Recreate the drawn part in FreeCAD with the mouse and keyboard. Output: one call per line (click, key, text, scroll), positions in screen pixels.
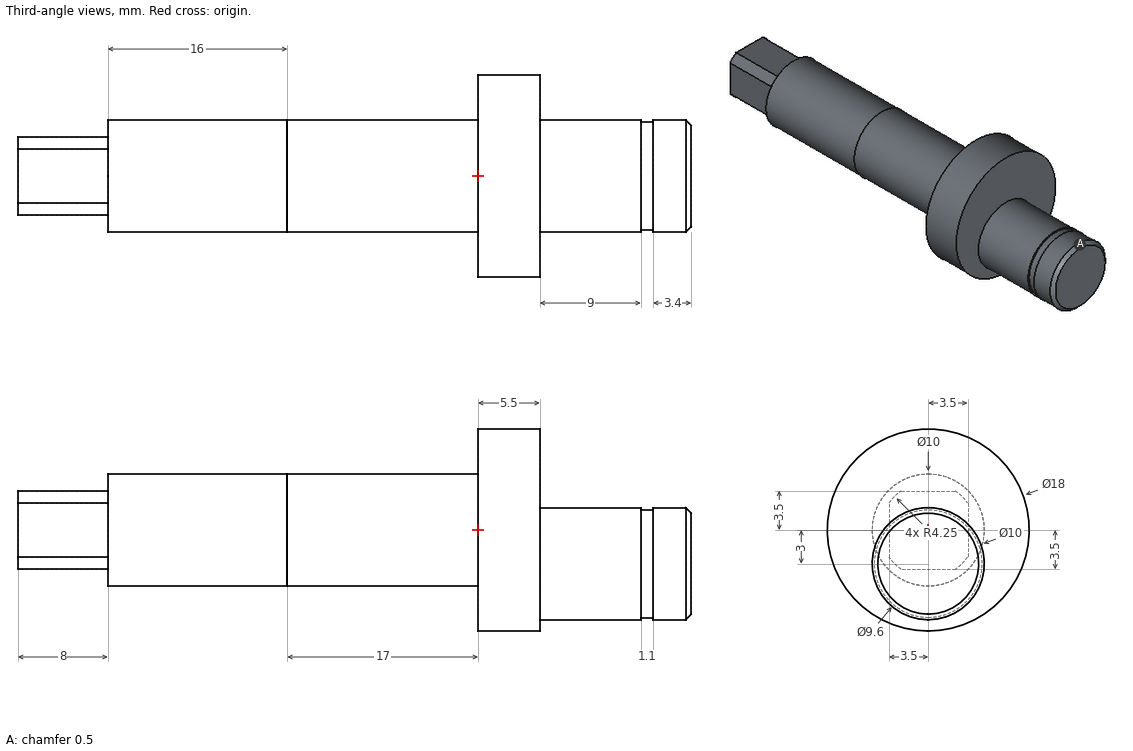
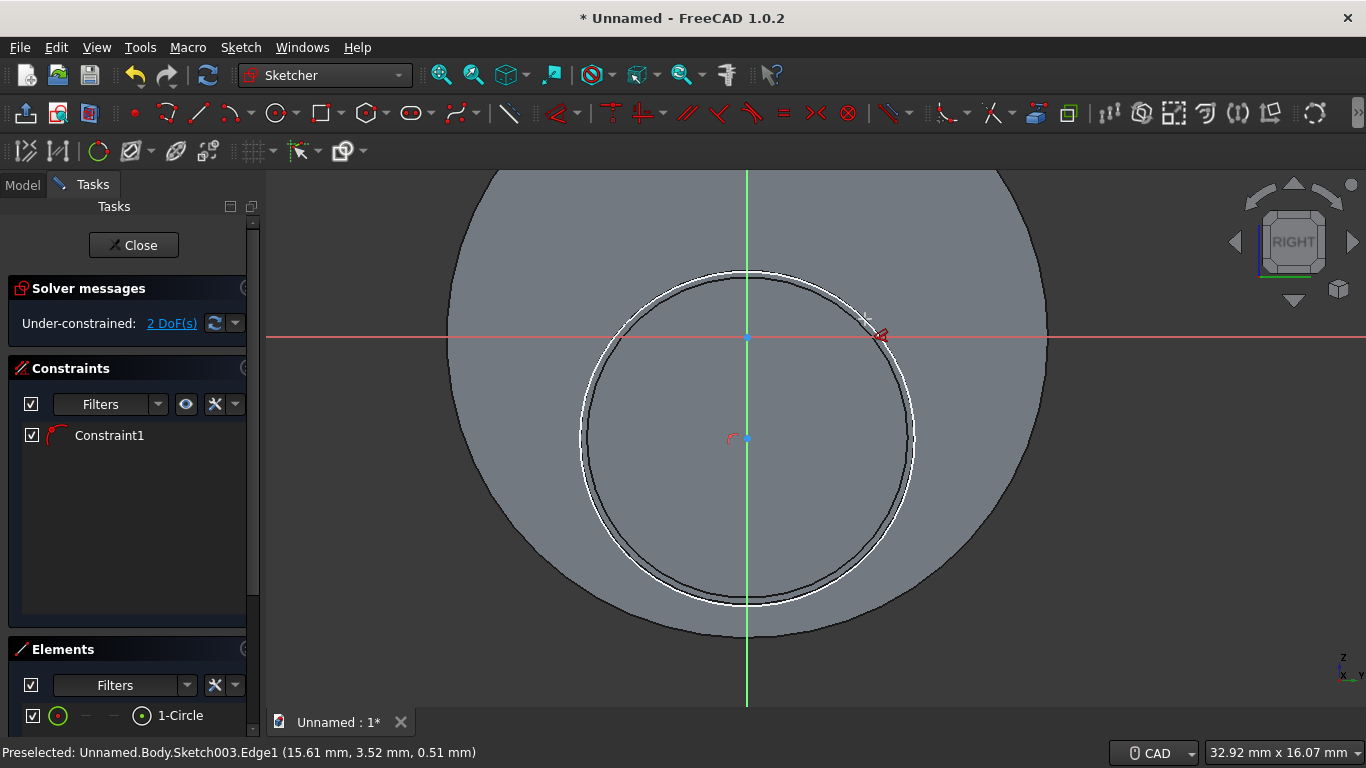
click(865, 320)
click(888, 297)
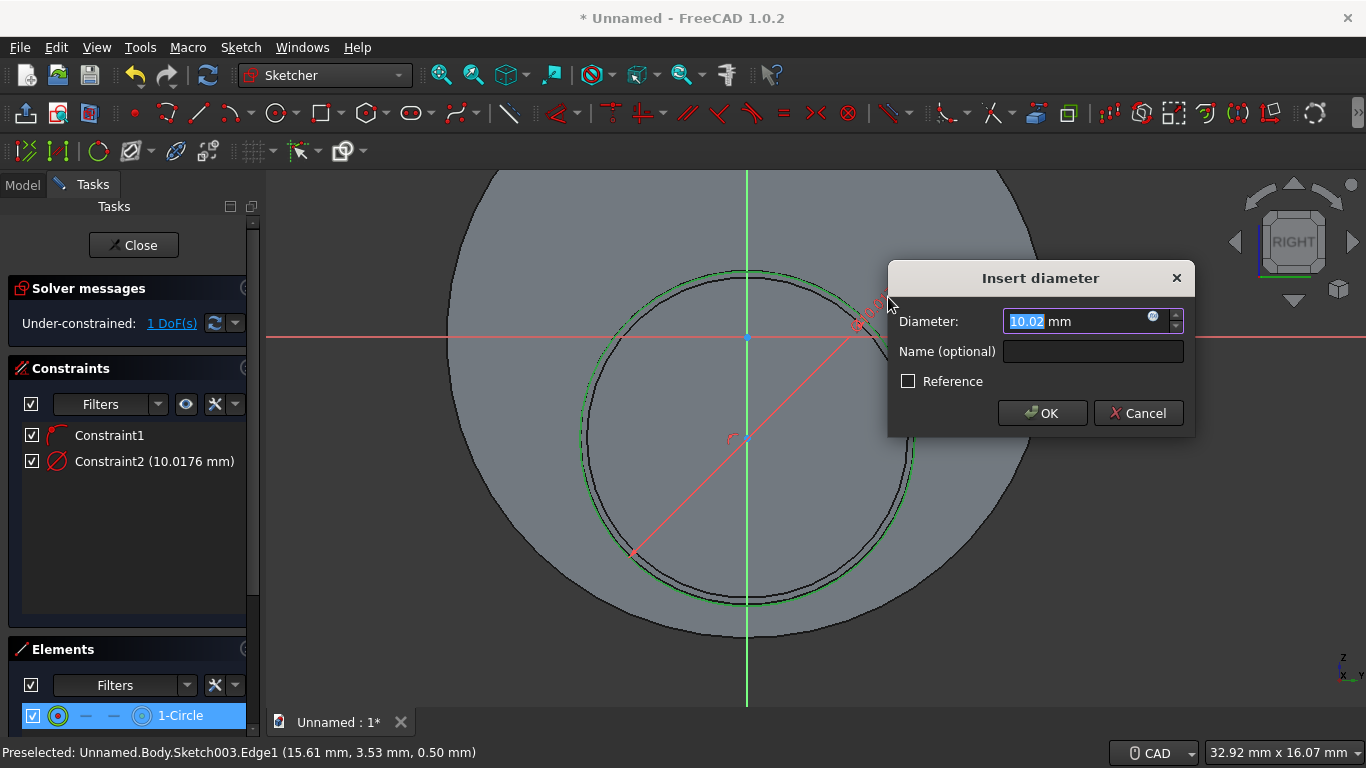
text(10)
key(Return)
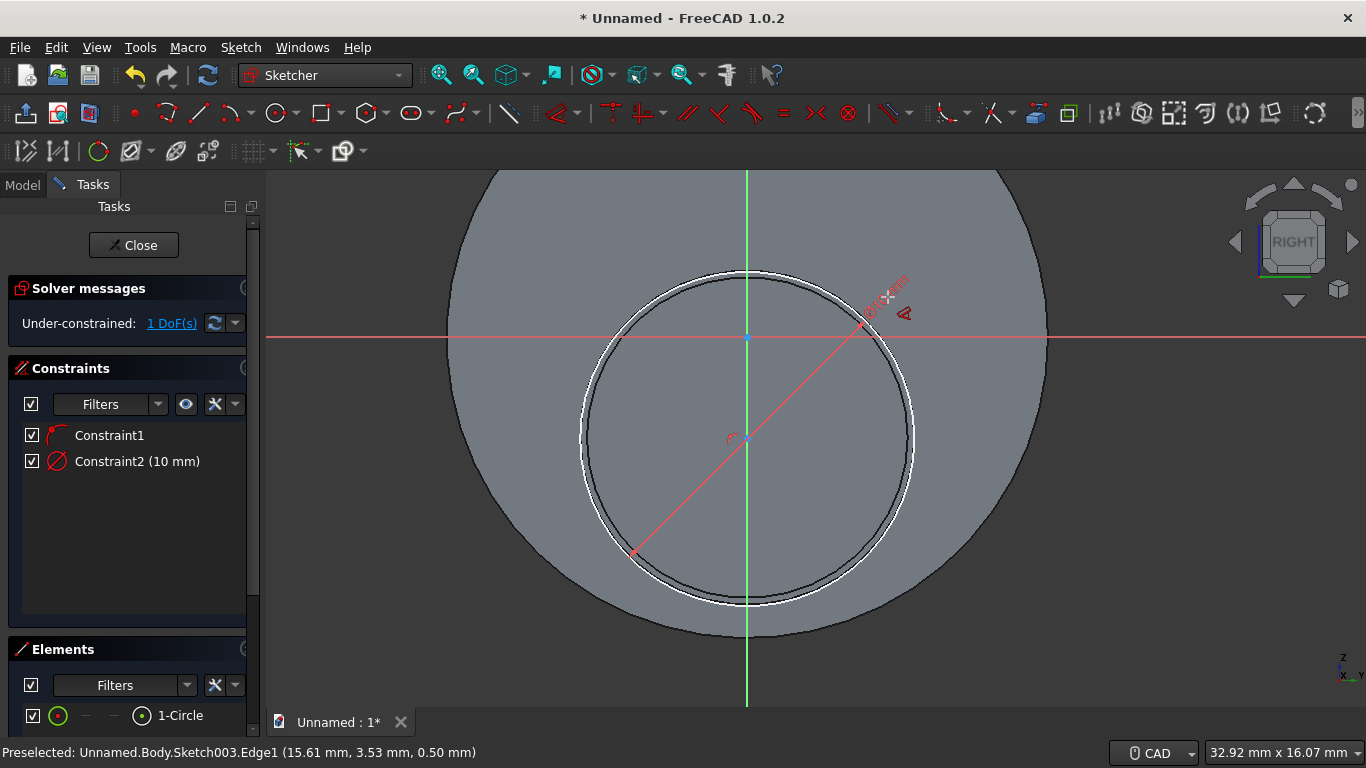
click(747, 439)
click(781, 388)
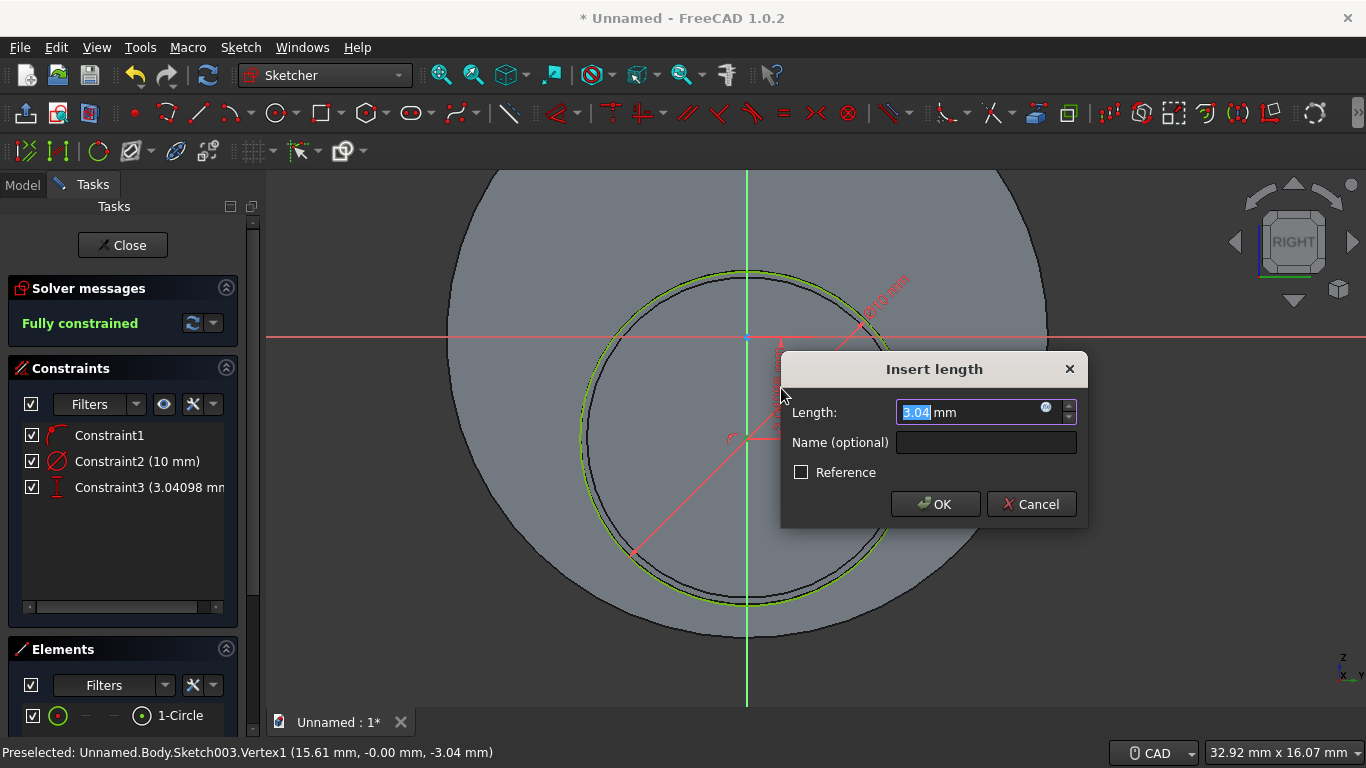
text(3)
key(Return)
key(Escape)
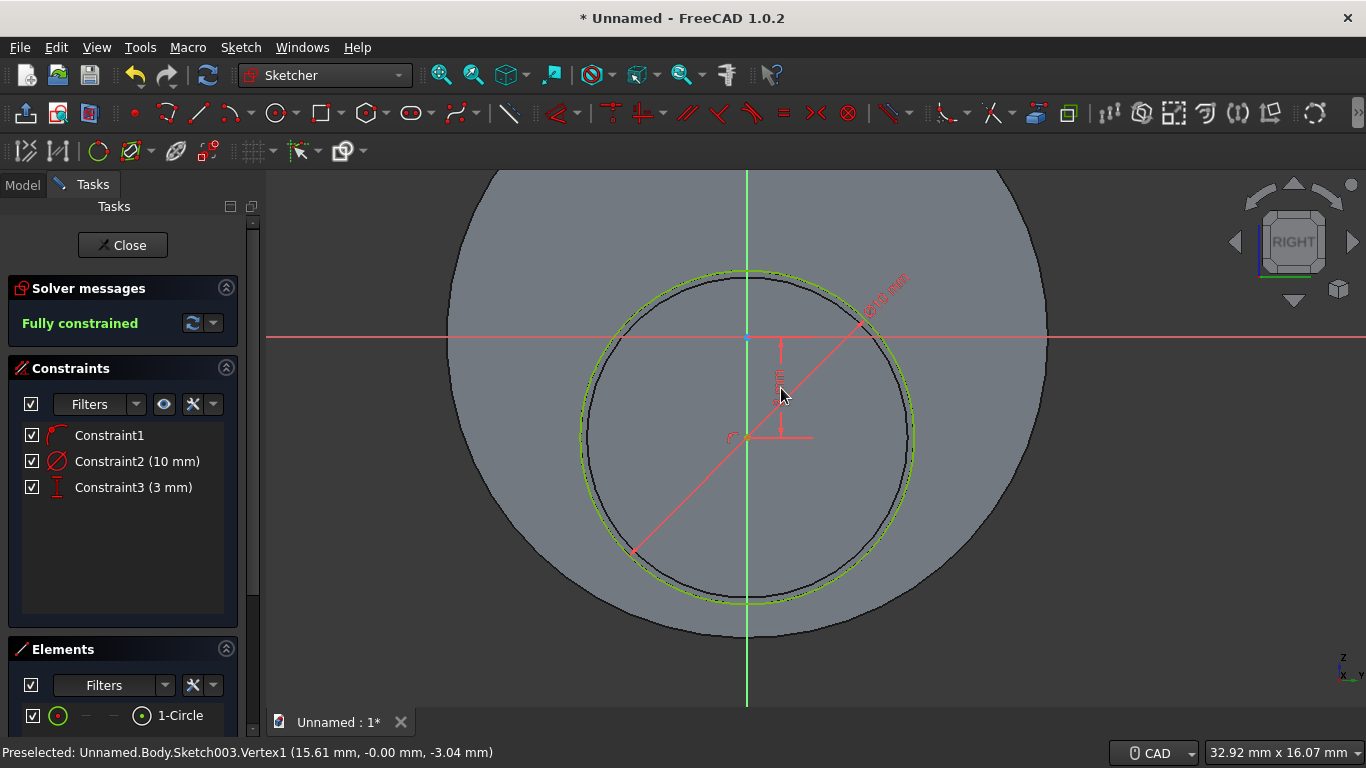
click(123, 245)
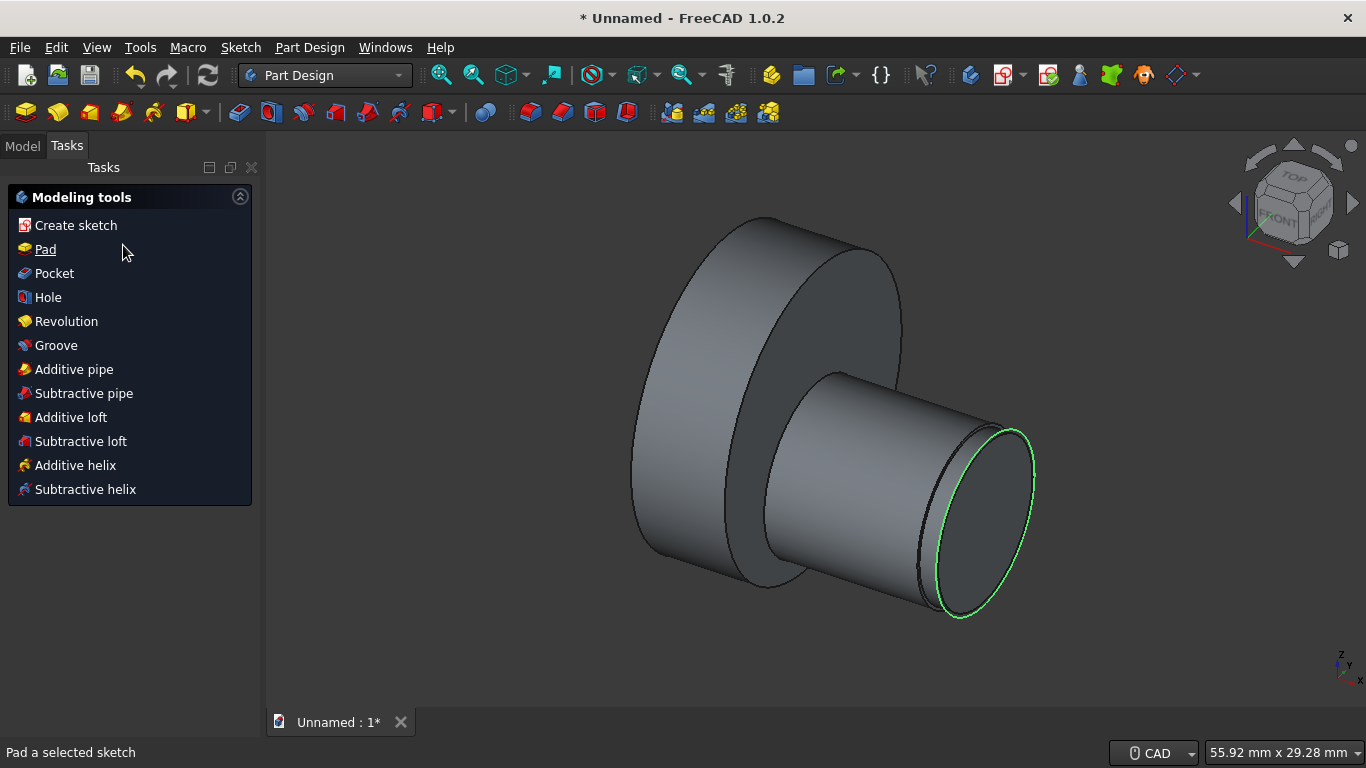
click(26, 112)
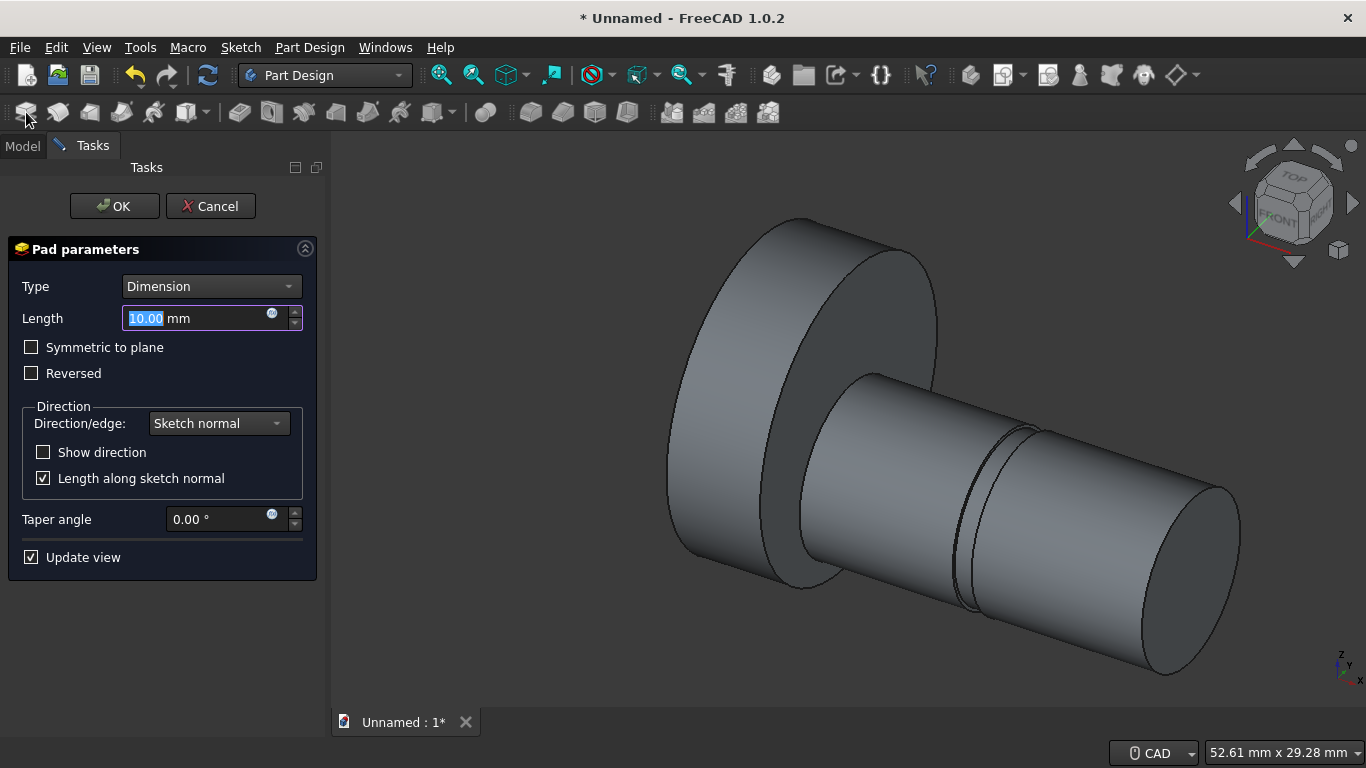
text(3.4)
key(Tab)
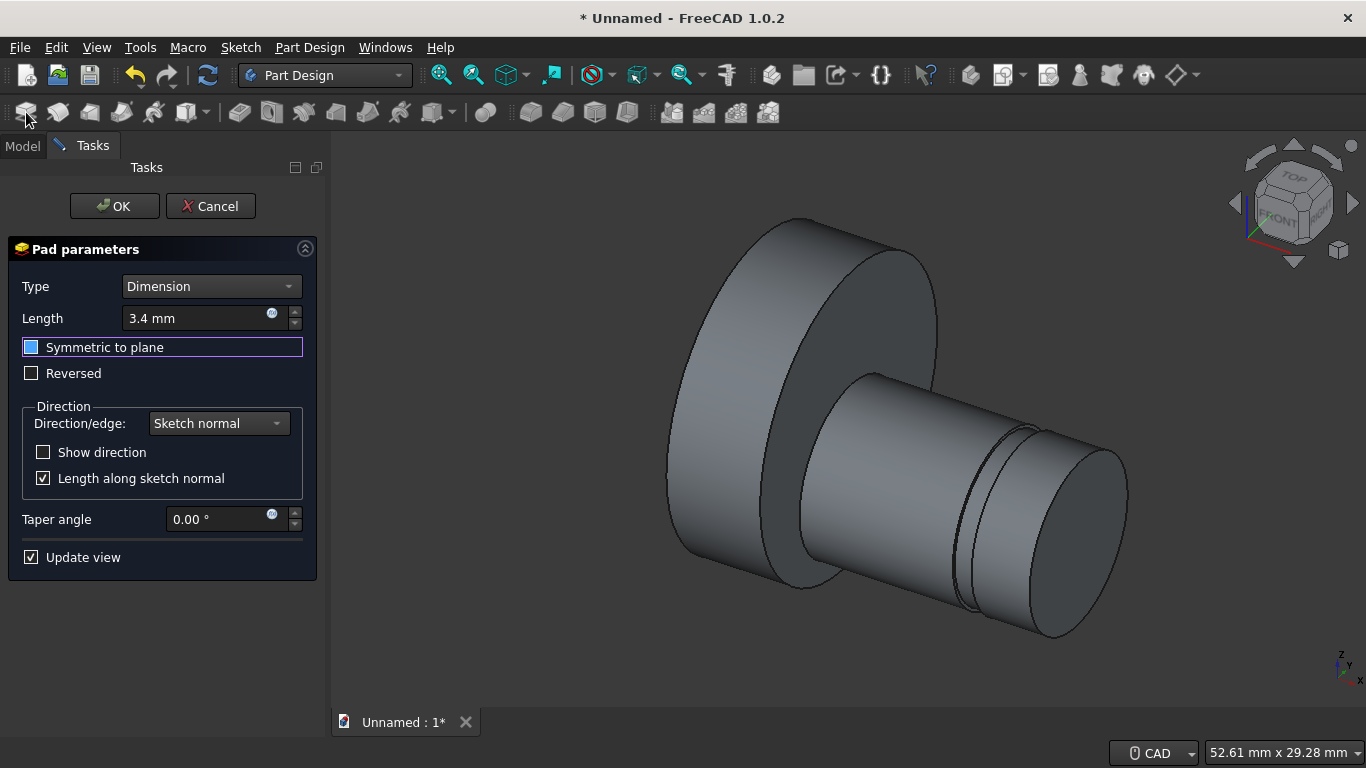
click(115, 206)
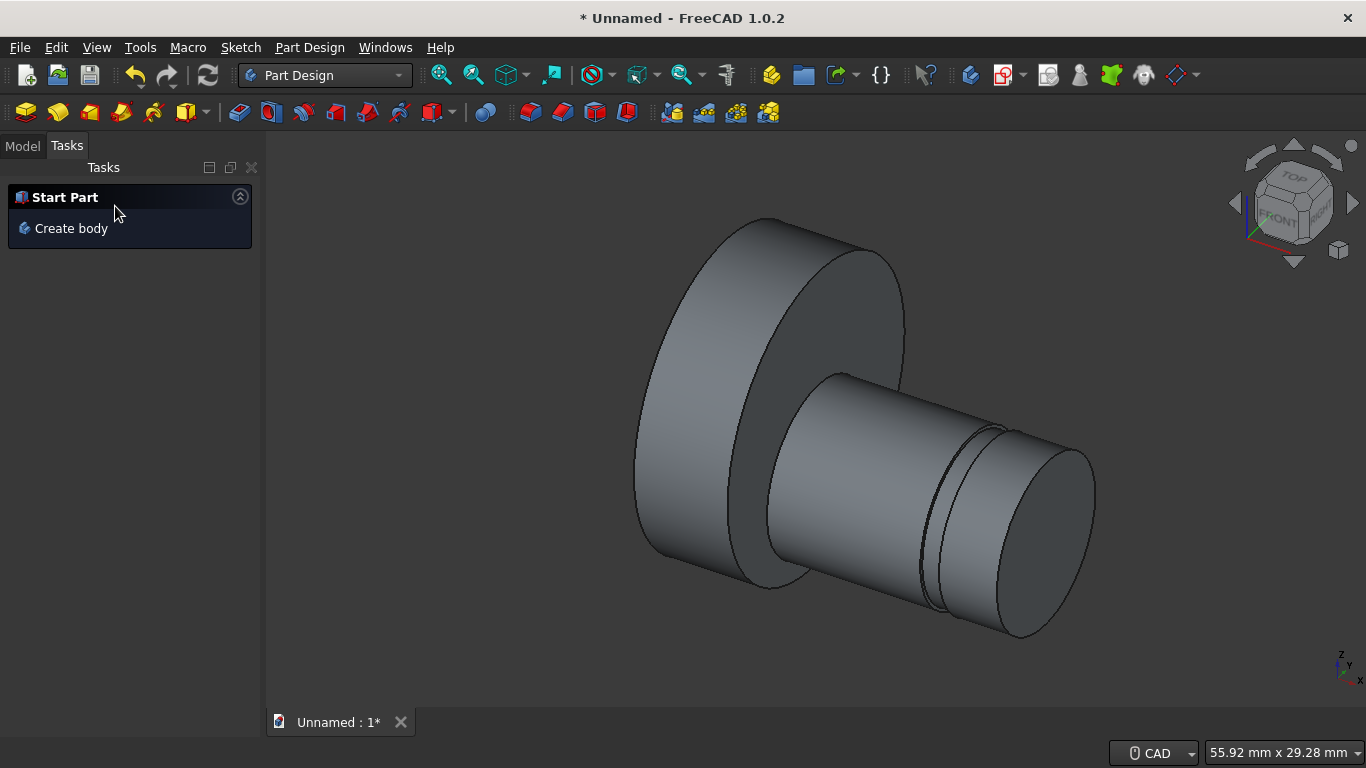
key(v)
key(f)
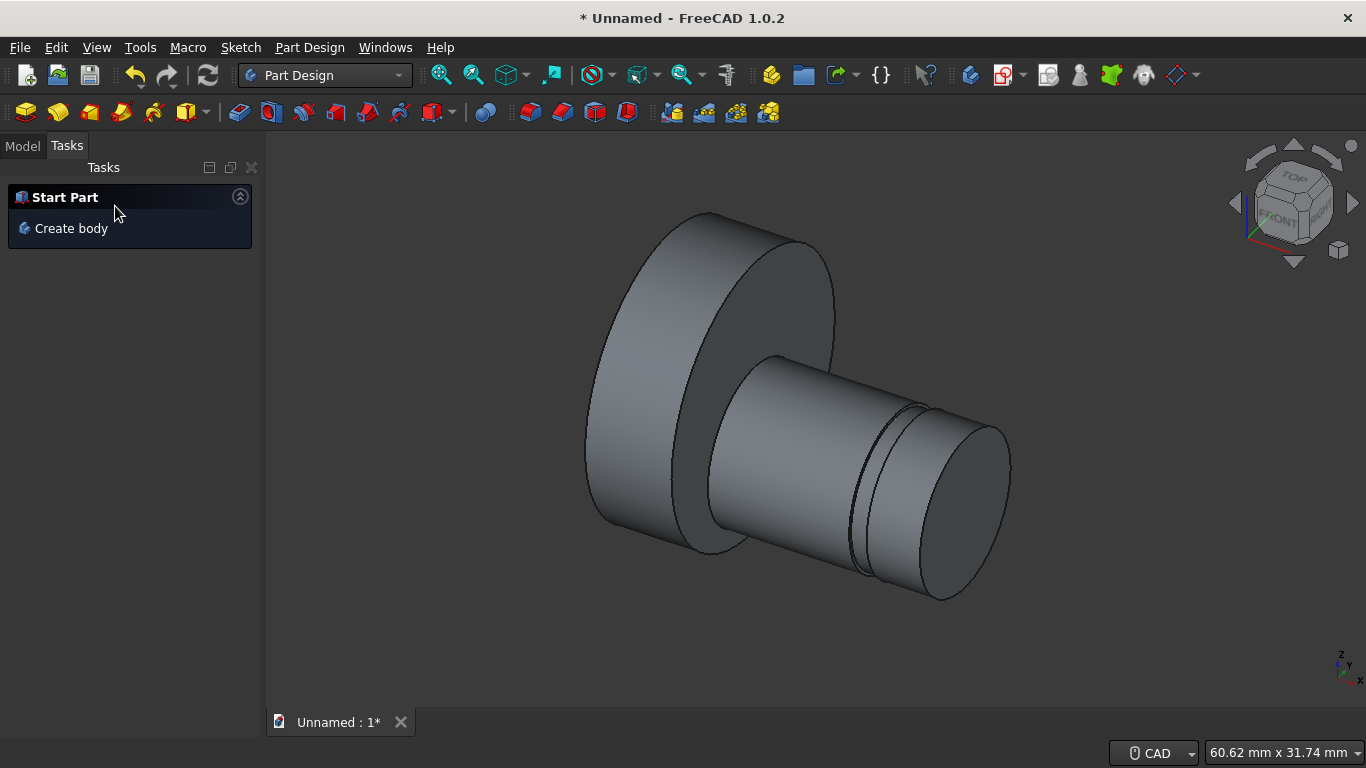
click(920, 557)